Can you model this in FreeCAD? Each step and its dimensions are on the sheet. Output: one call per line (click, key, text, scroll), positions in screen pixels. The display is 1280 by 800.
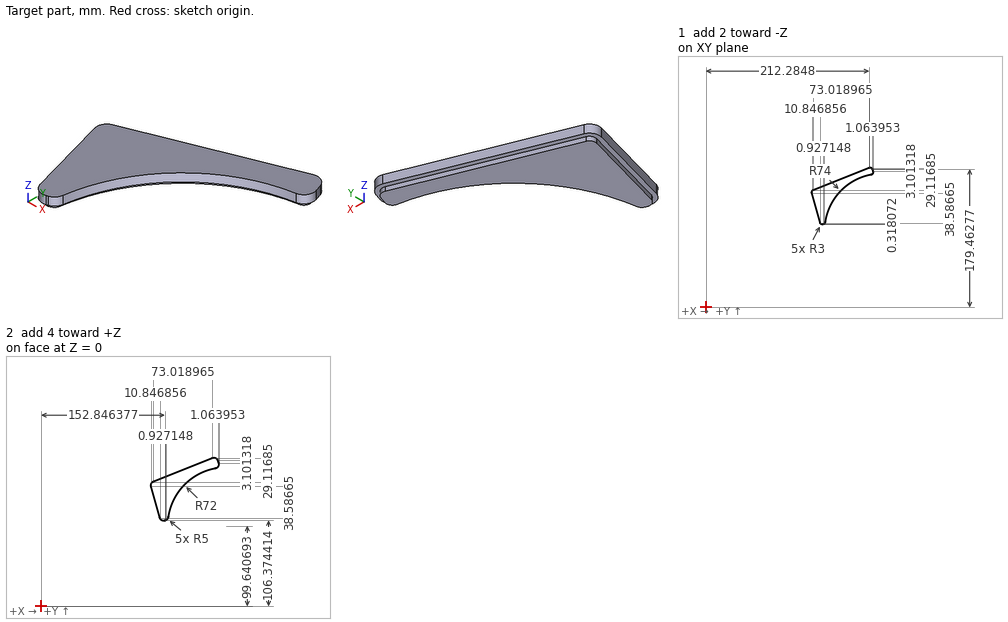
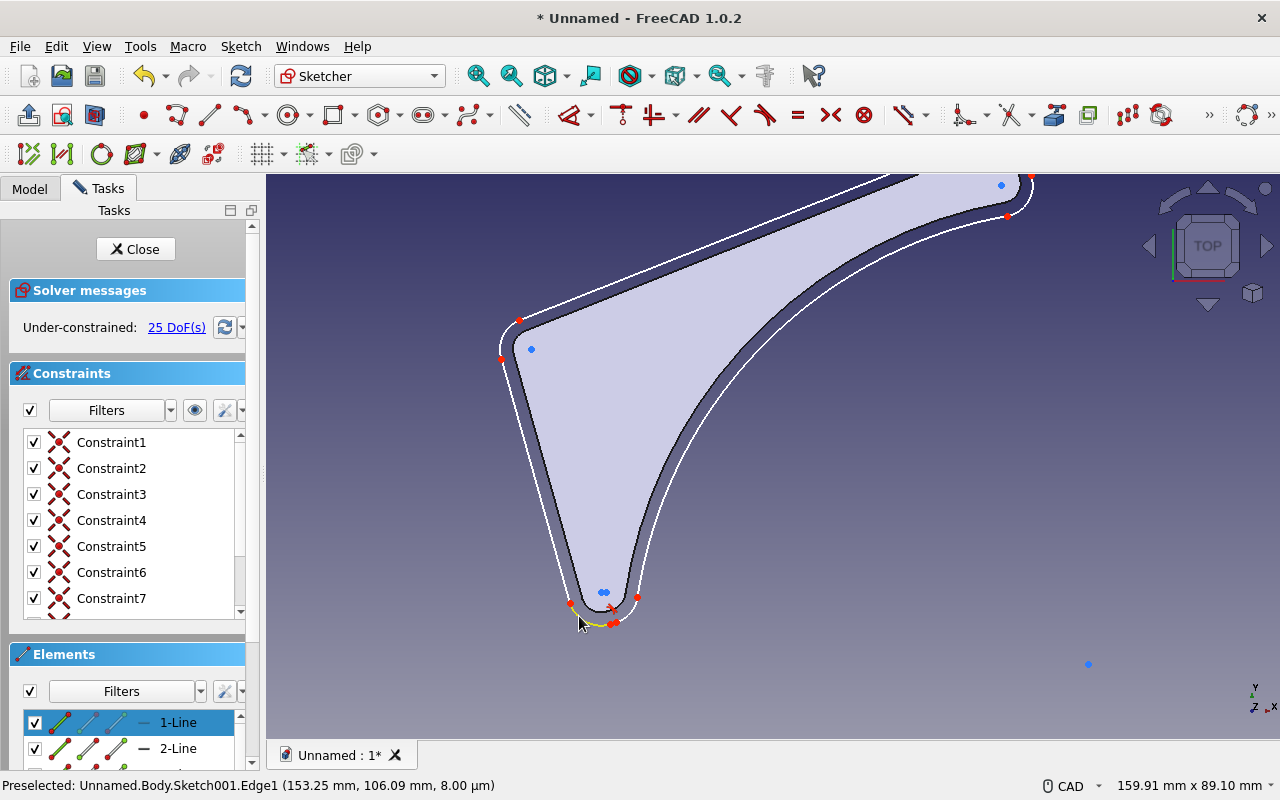
click(578, 616)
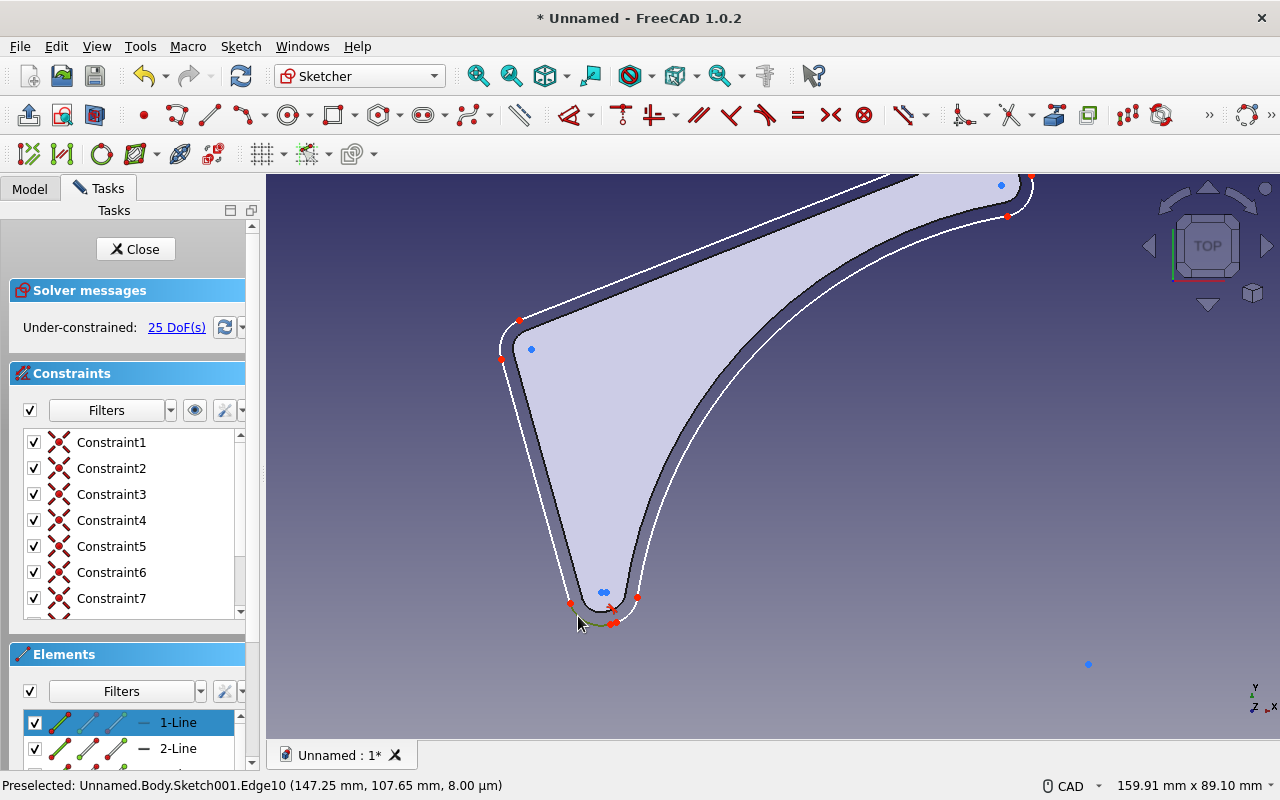
click(765, 116)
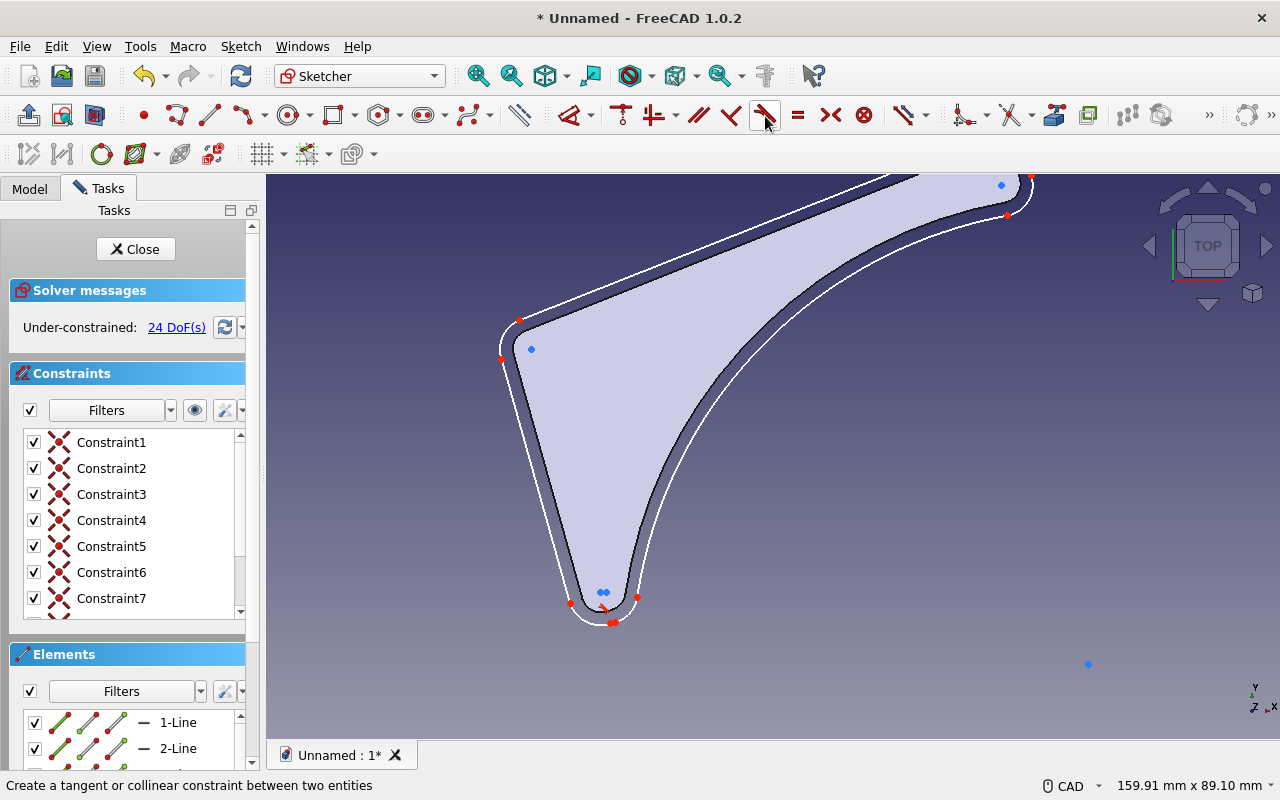
scroll(578, 614, down, 2)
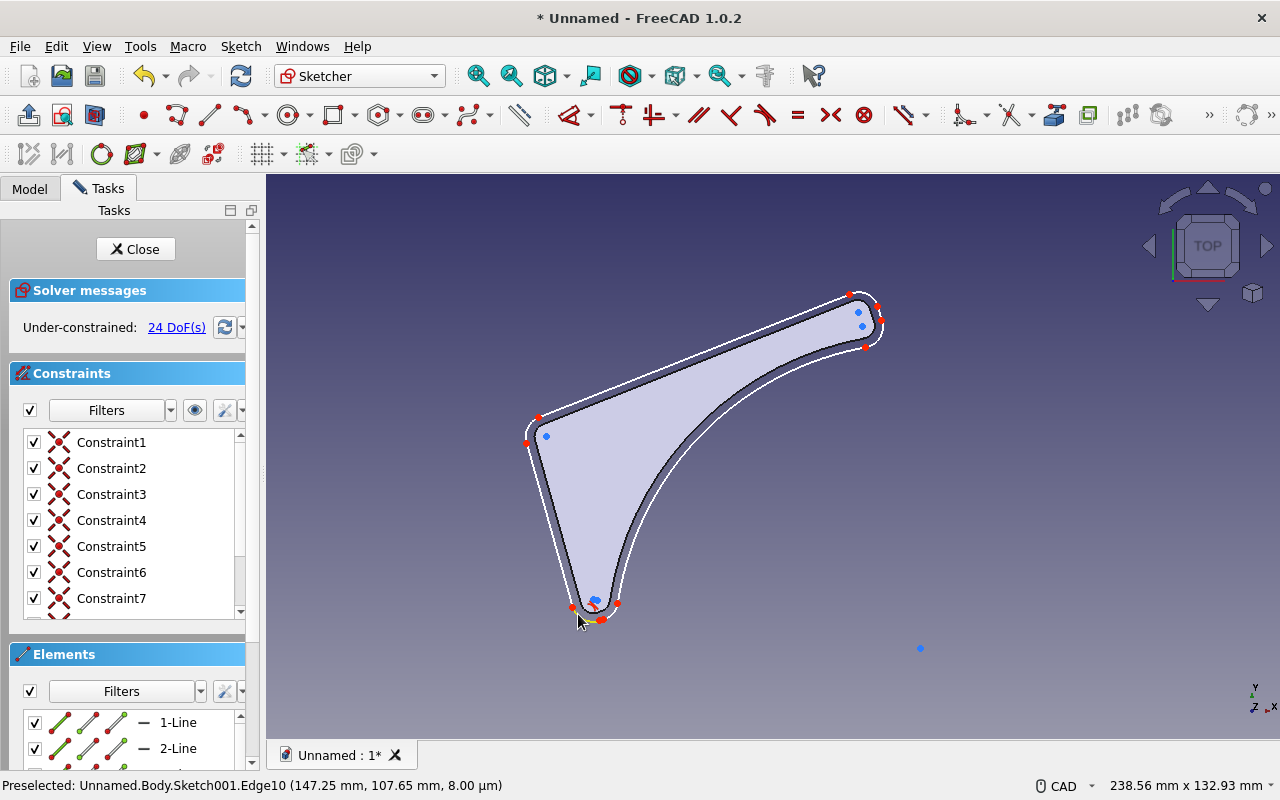
scroll(880, 313, up, 4)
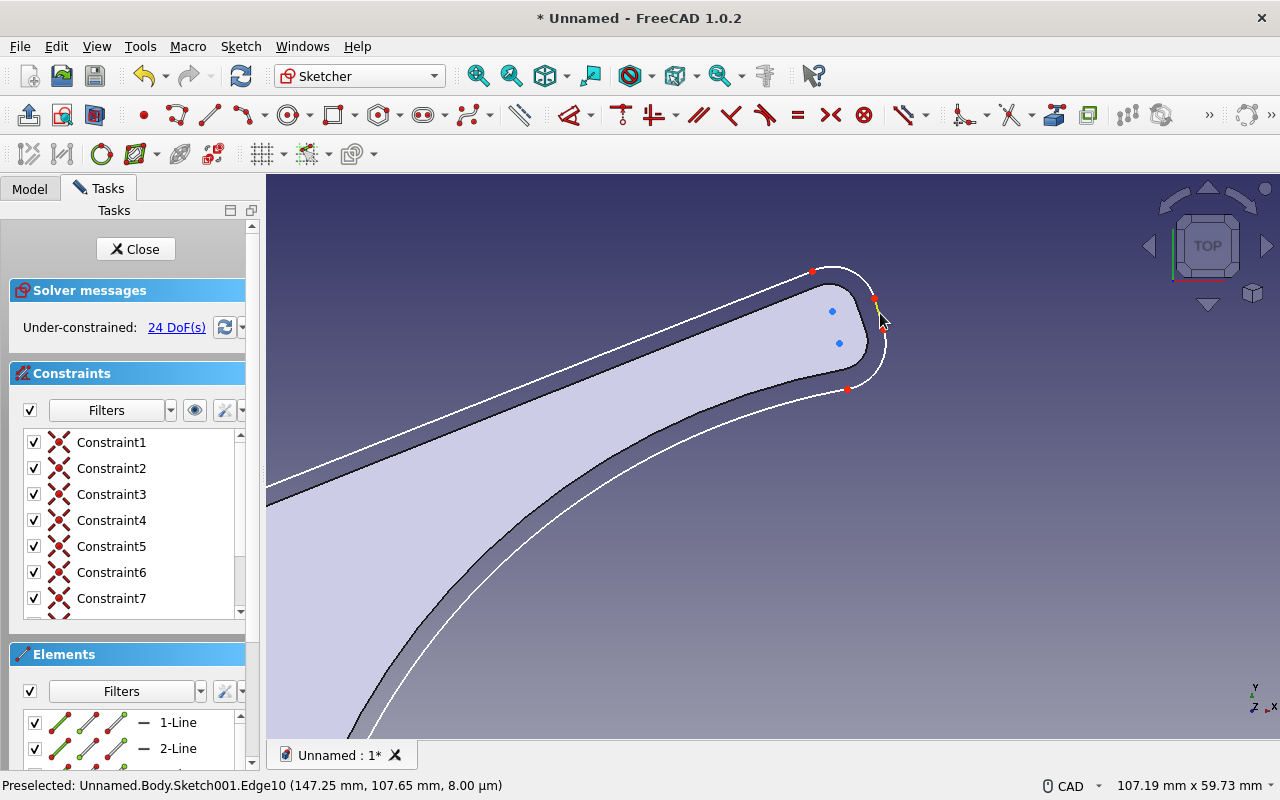
click(879, 314)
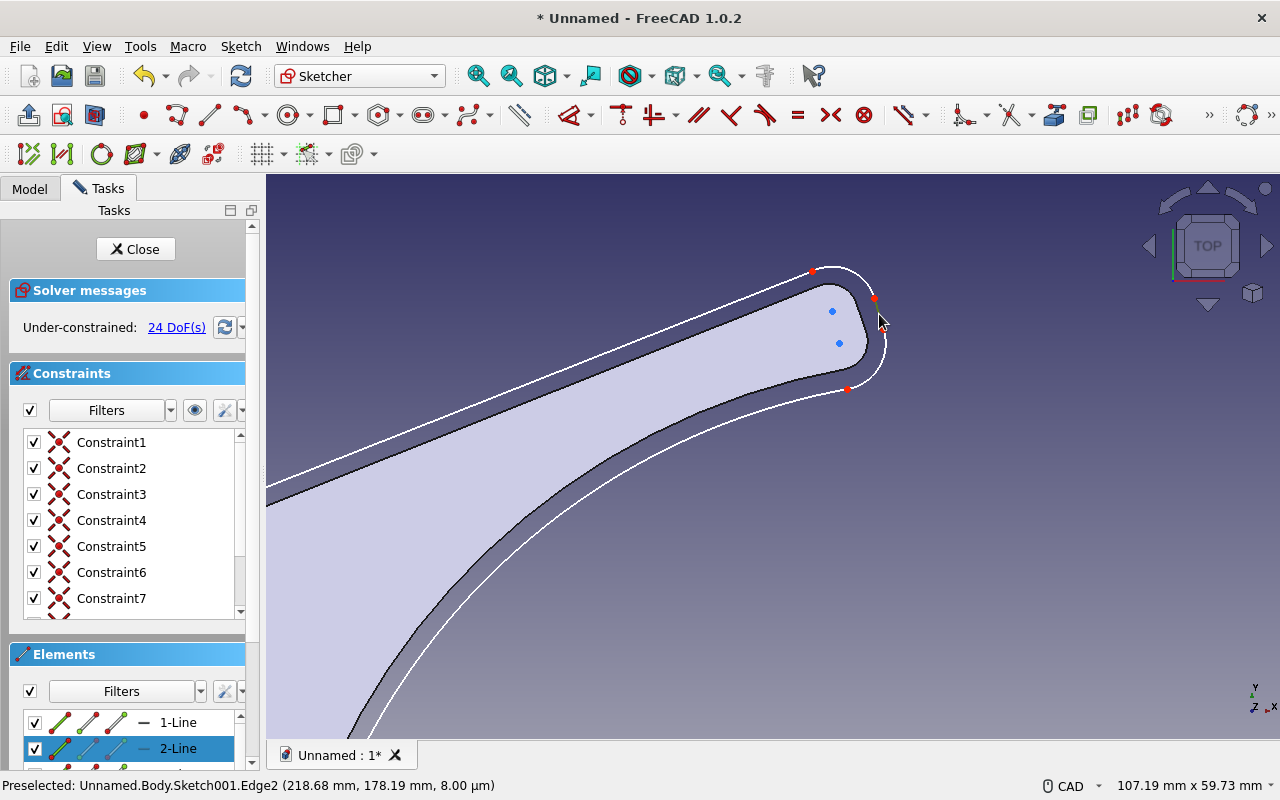
click(869, 379)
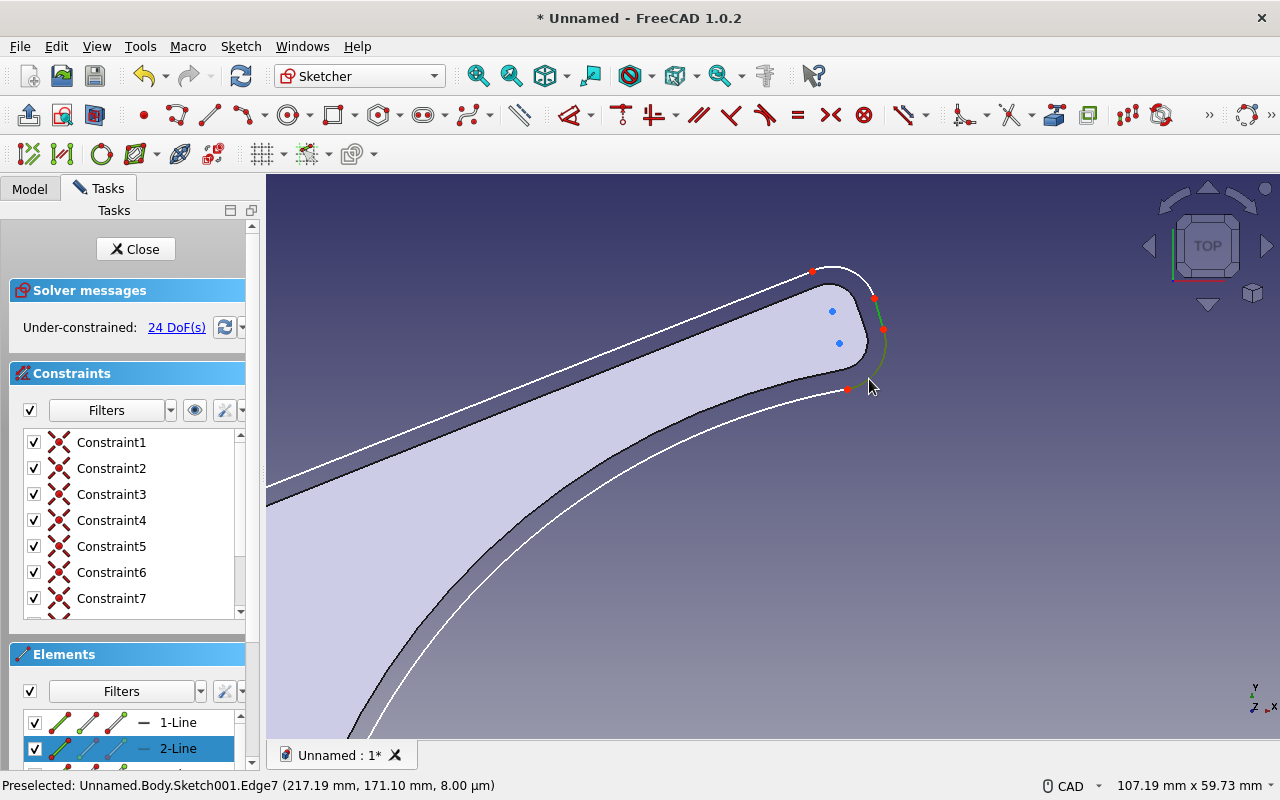
click(765, 116)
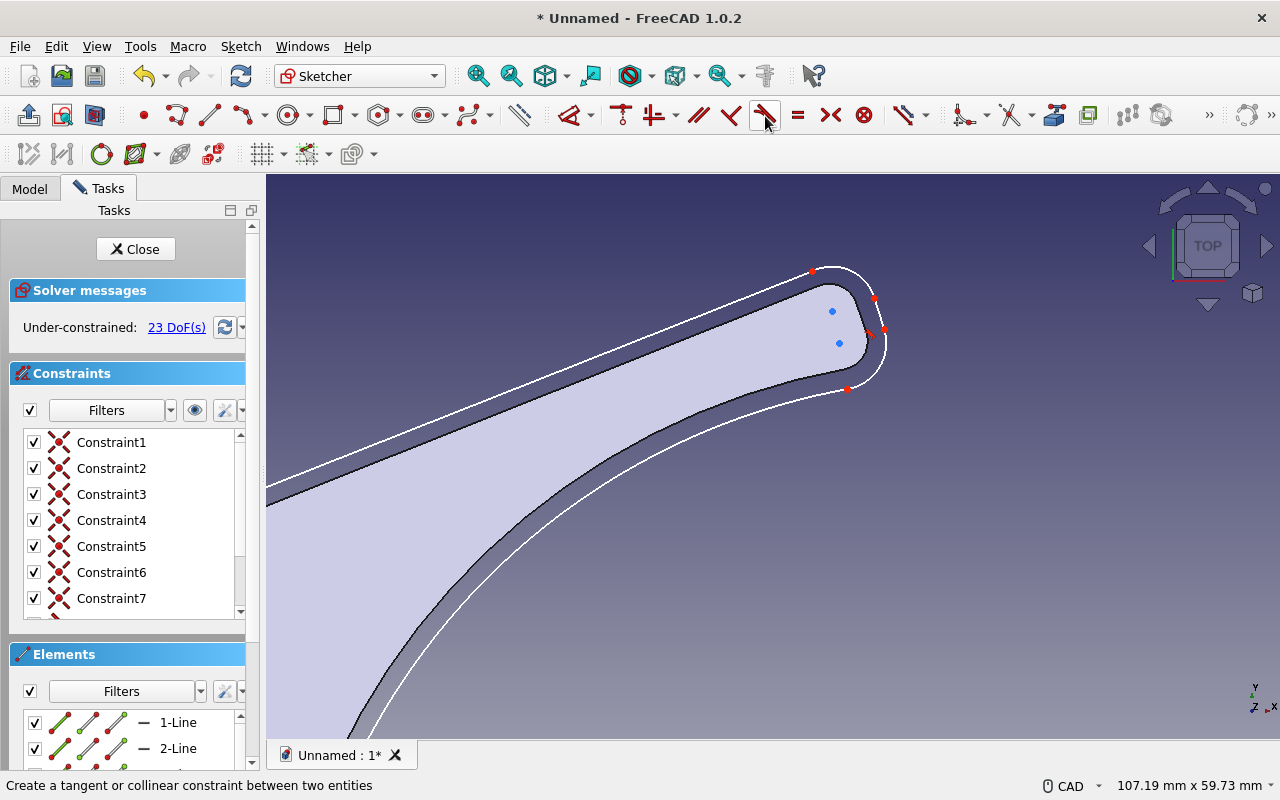
scroll(881, 320, up, 2)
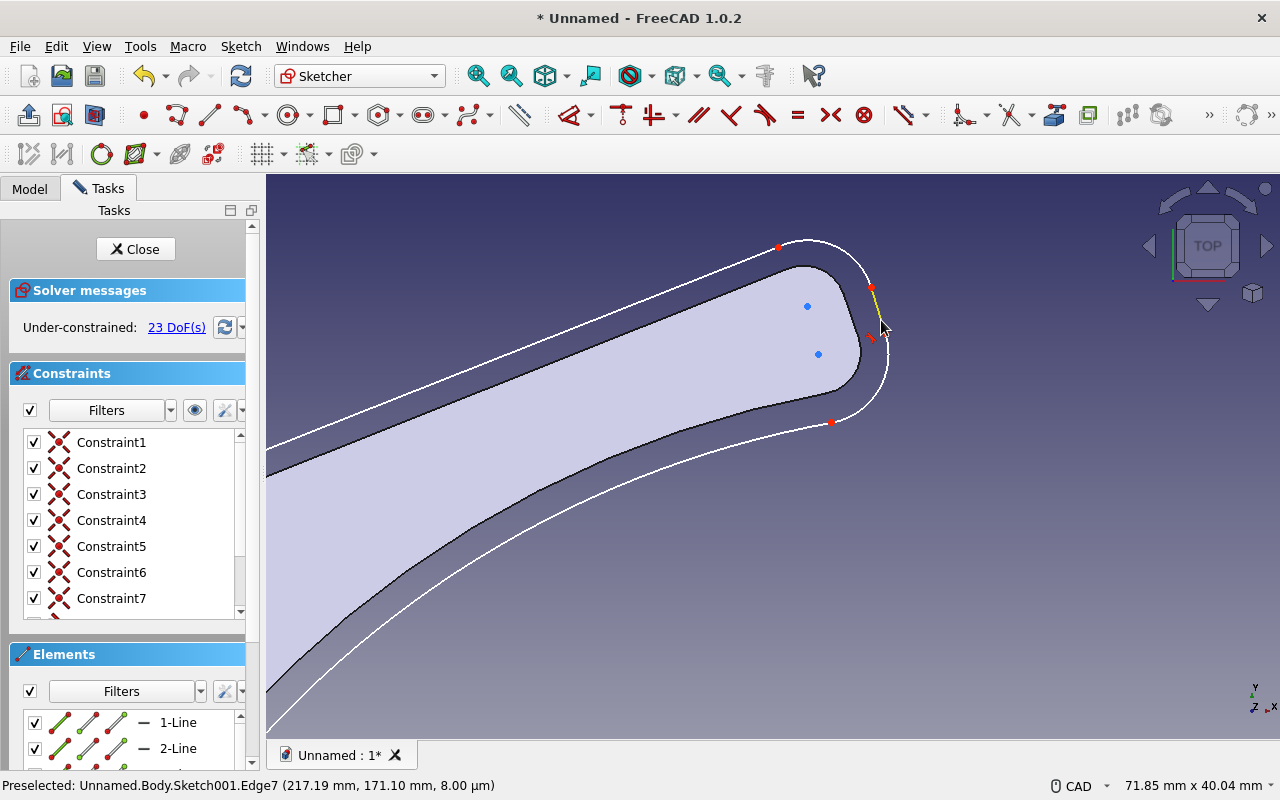
click(881, 320)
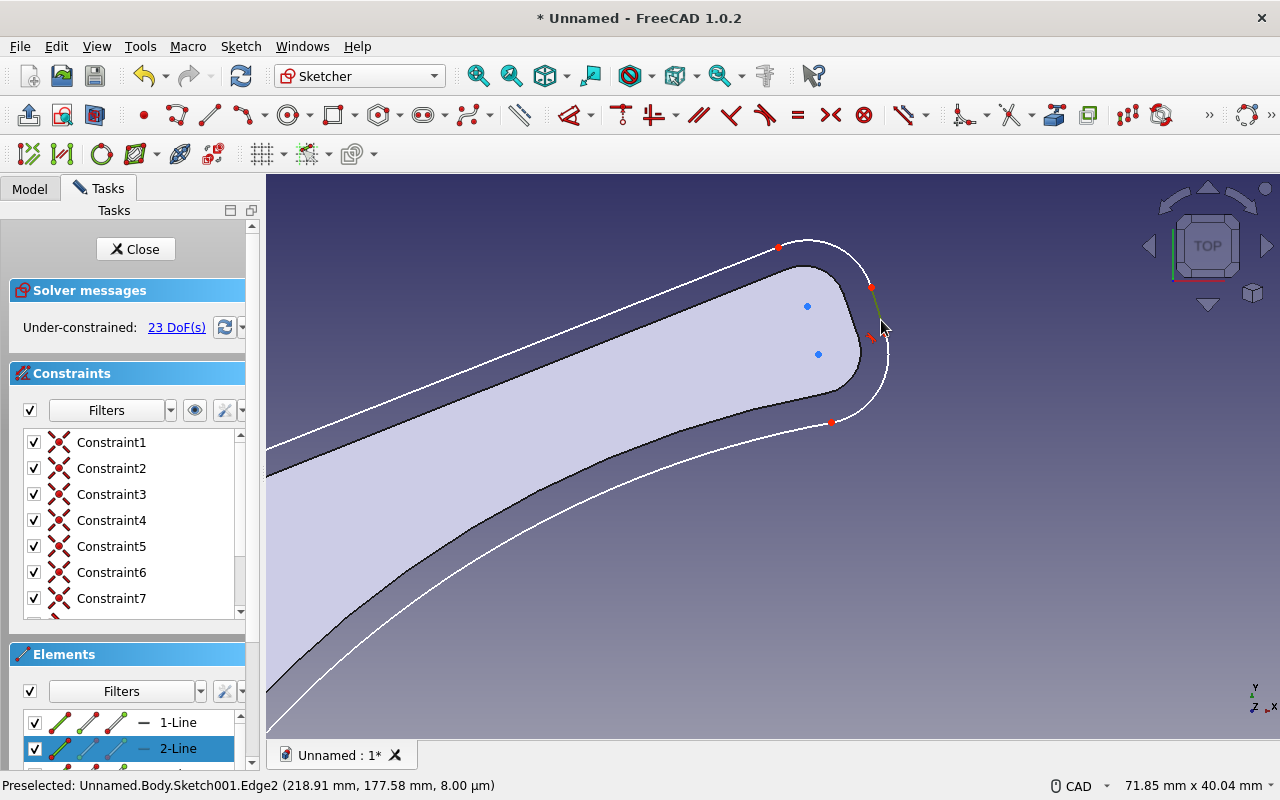
click(853, 258)